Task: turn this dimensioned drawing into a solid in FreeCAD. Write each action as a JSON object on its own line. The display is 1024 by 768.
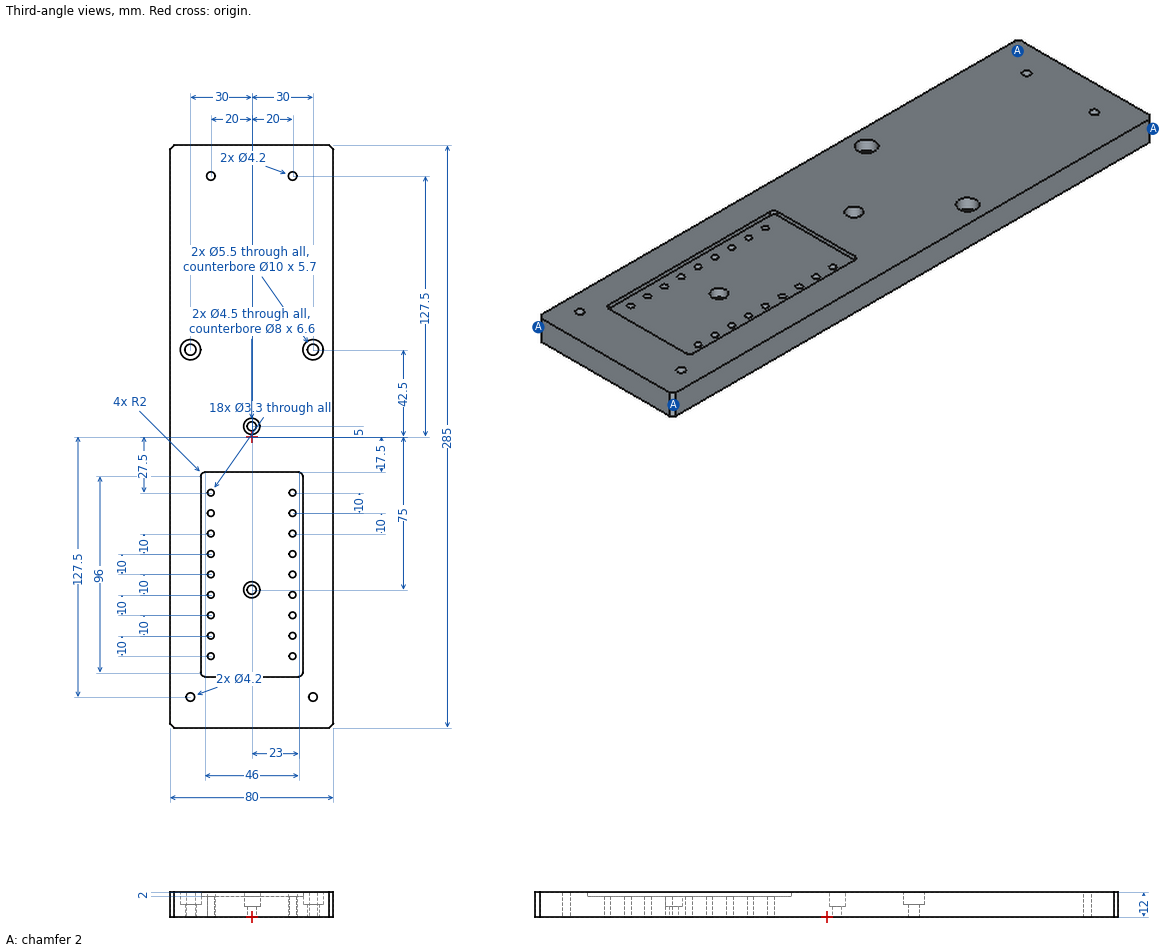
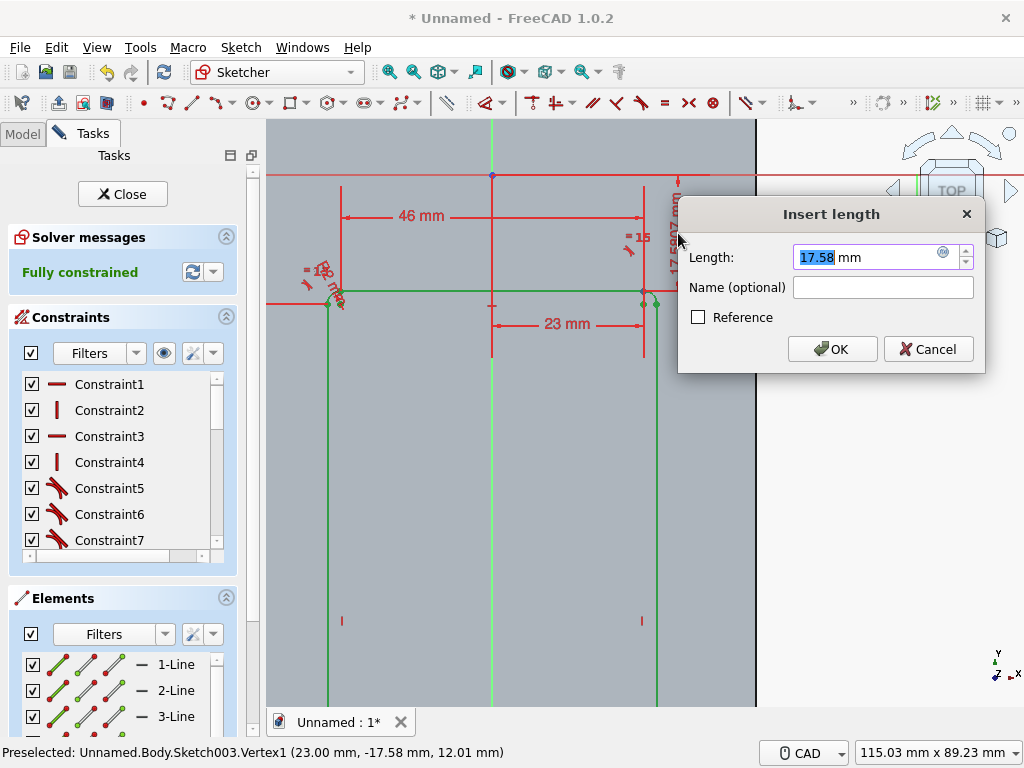
{"action": "type", "text": "17.5"}
{"action": "key", "text": "Return"}
{"action": "key", "text": "Escape"}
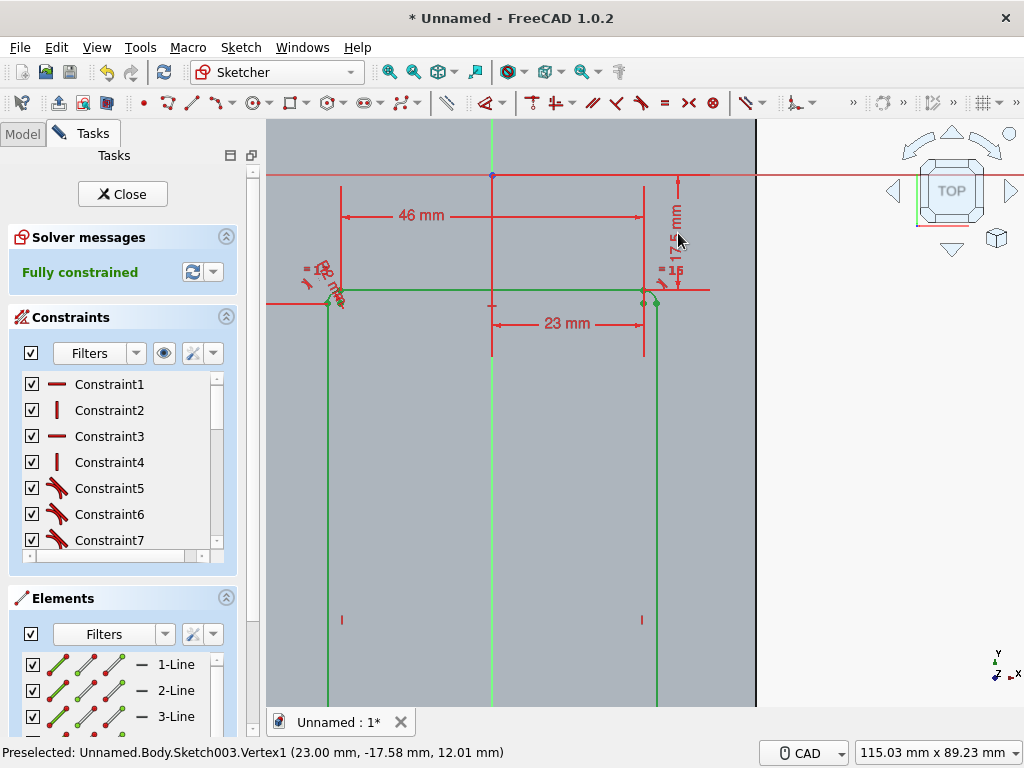
{"action": "left_click", "coordinate": [123, 194]}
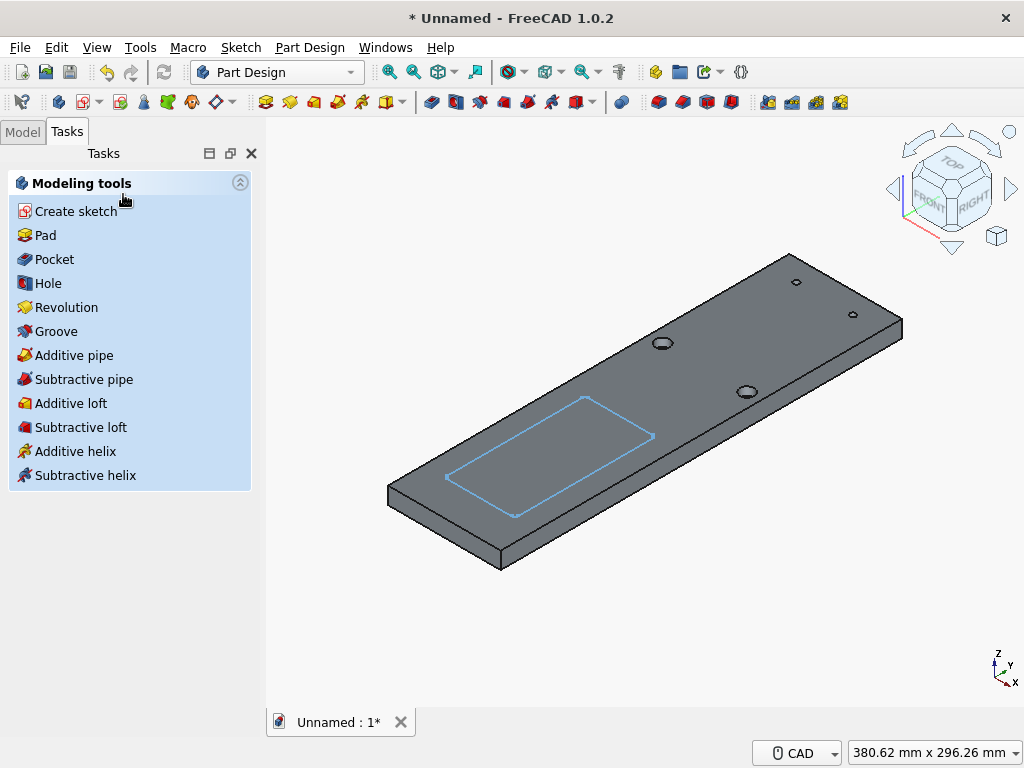
{"action": "left_click", "coordinate": [432, 102]}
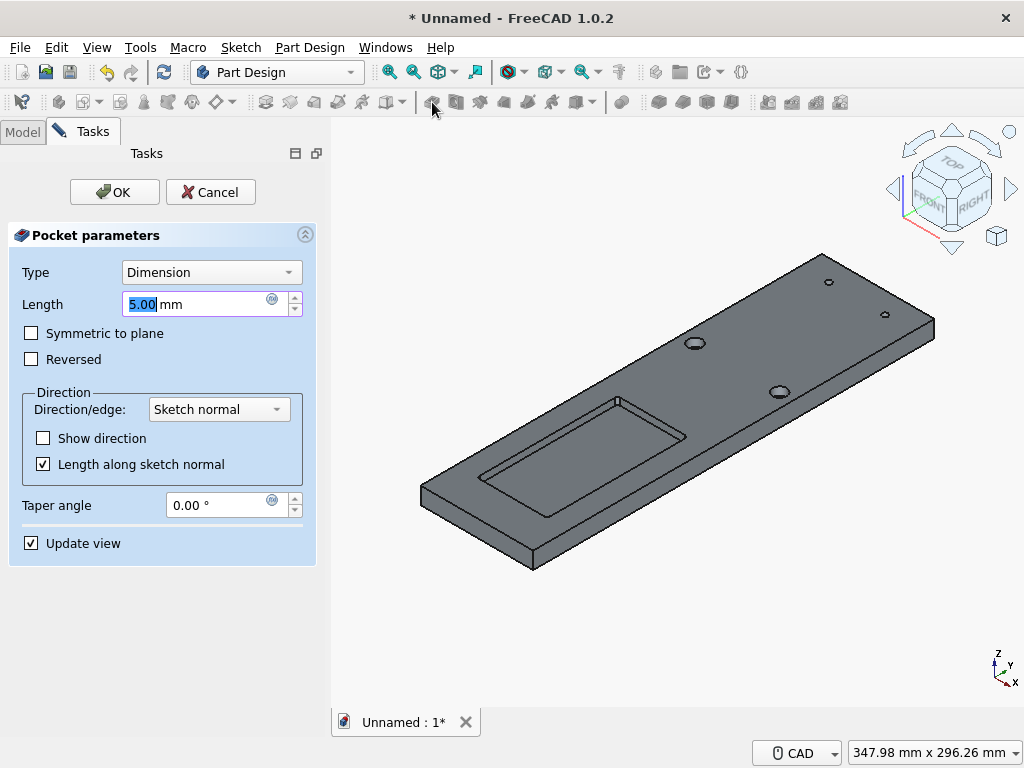
{"action": "type", "text": "2"}
{"action": "key", "text": "Tab"}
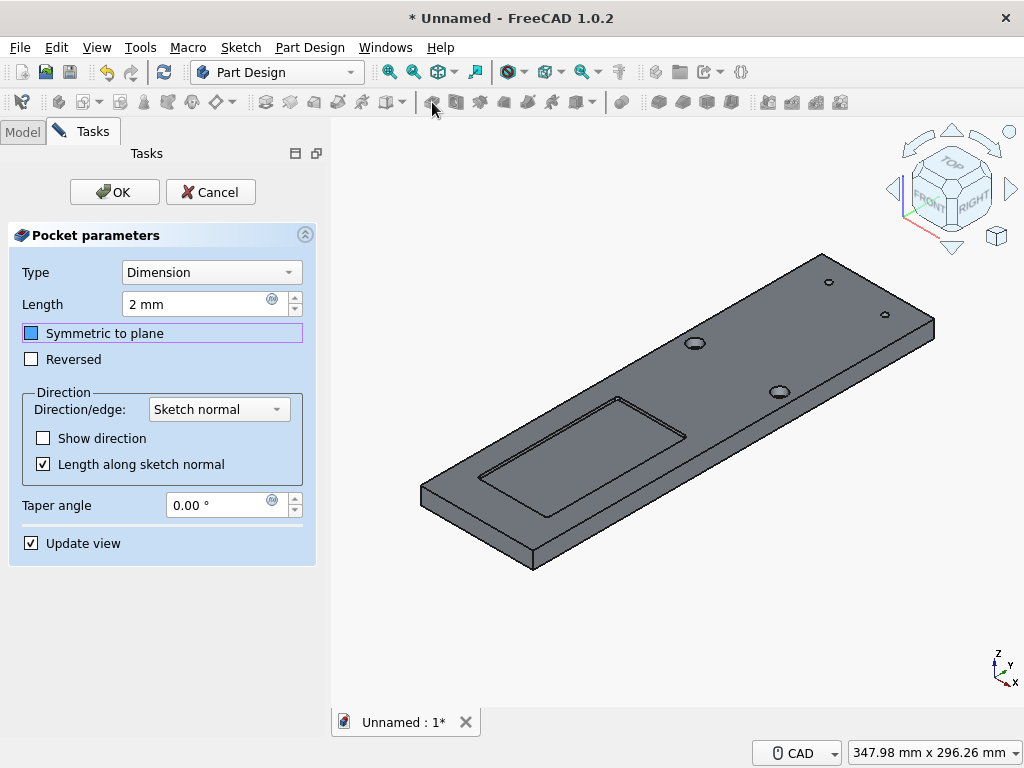
{"action": "left_click", "coordinate": [115, 192]}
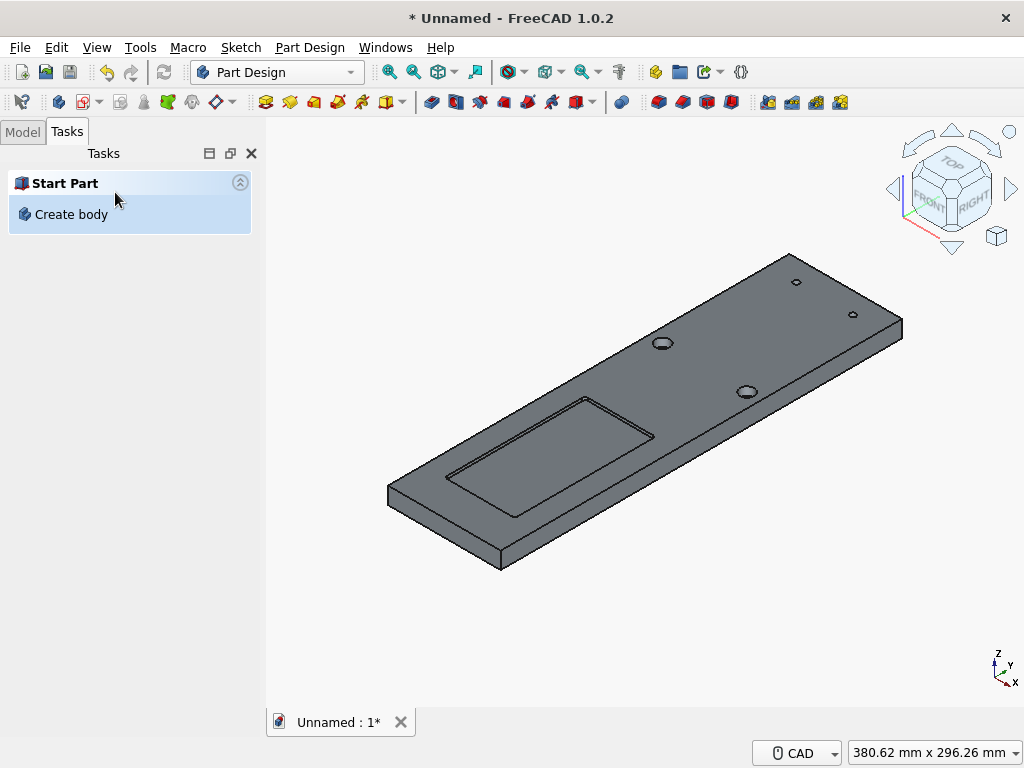
{"action": "left_click", "coordinate": [570, 448]}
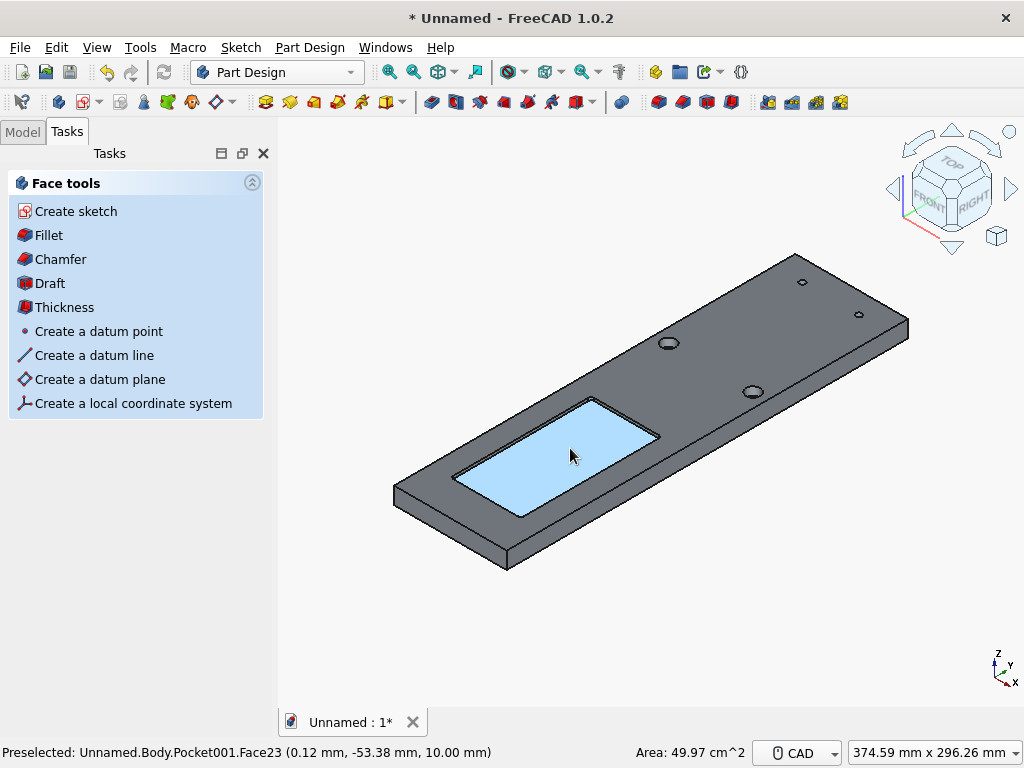
{"action": "left_click", "coordinate": [84, 102]}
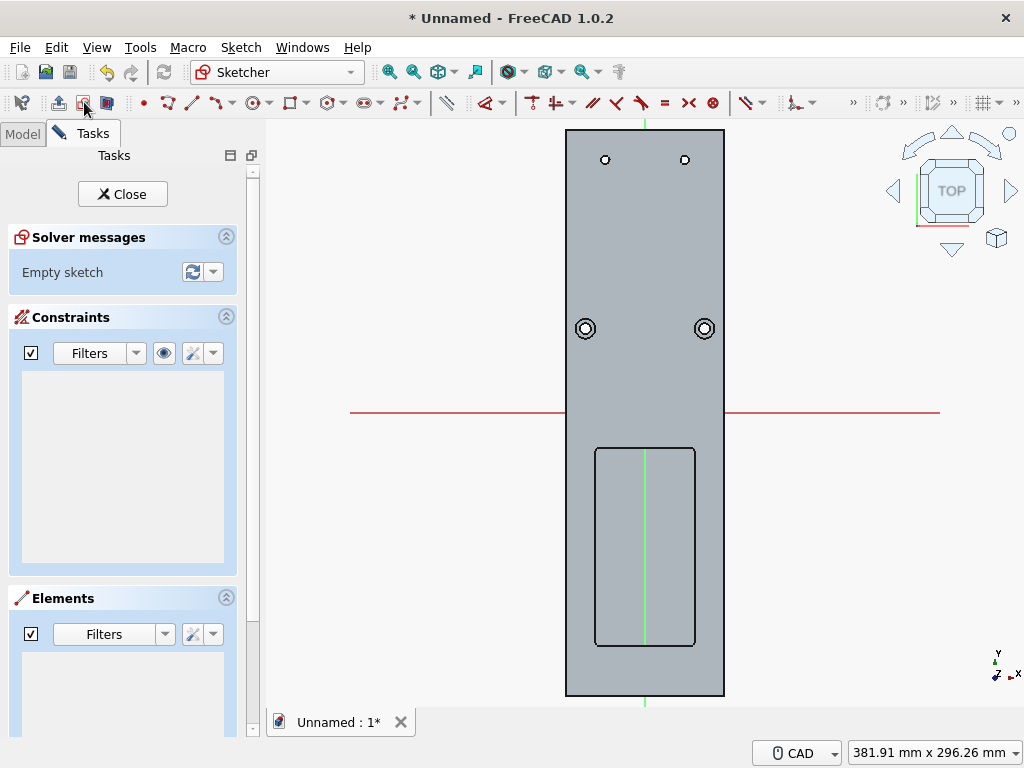
{"action": "key", "text": "q s"}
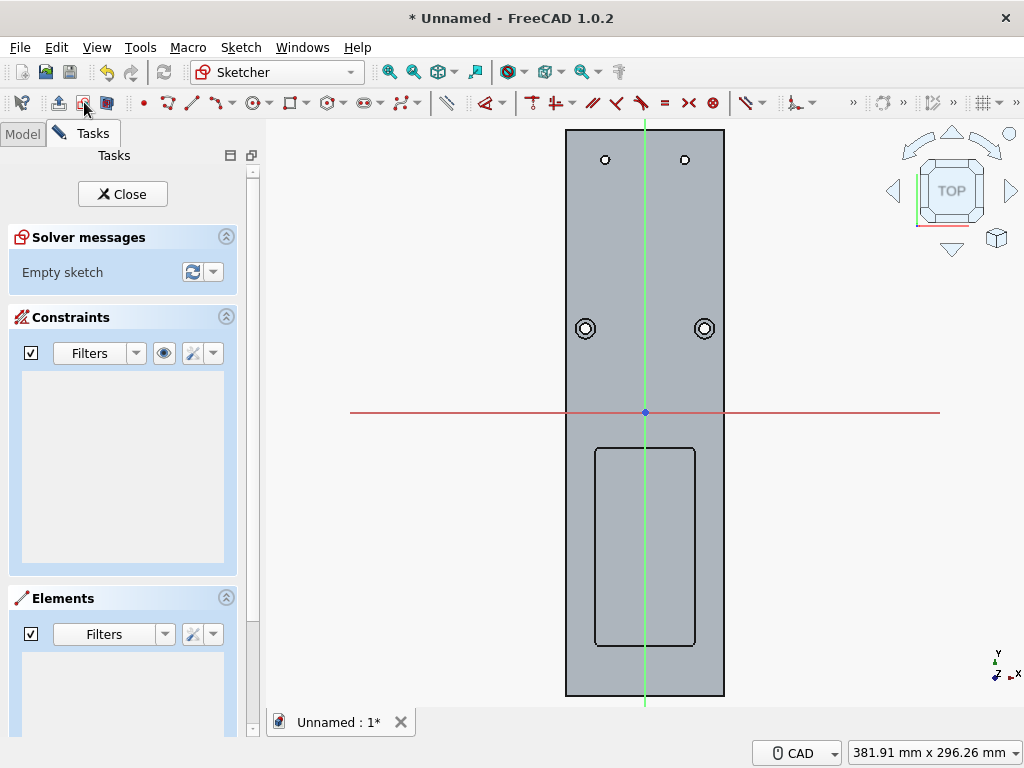
{"action": "scroll", "coordinate": [728, 653], "scroll_direction": "up", "scroll_amount": 3}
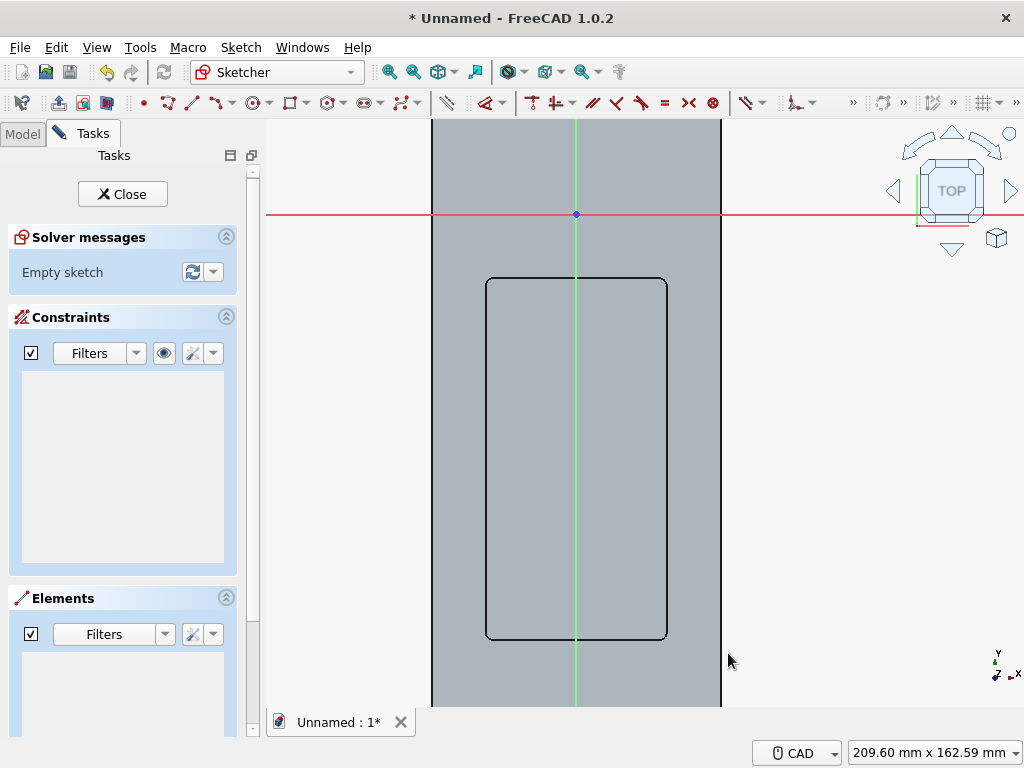
{"action": "key", "text": "g c"}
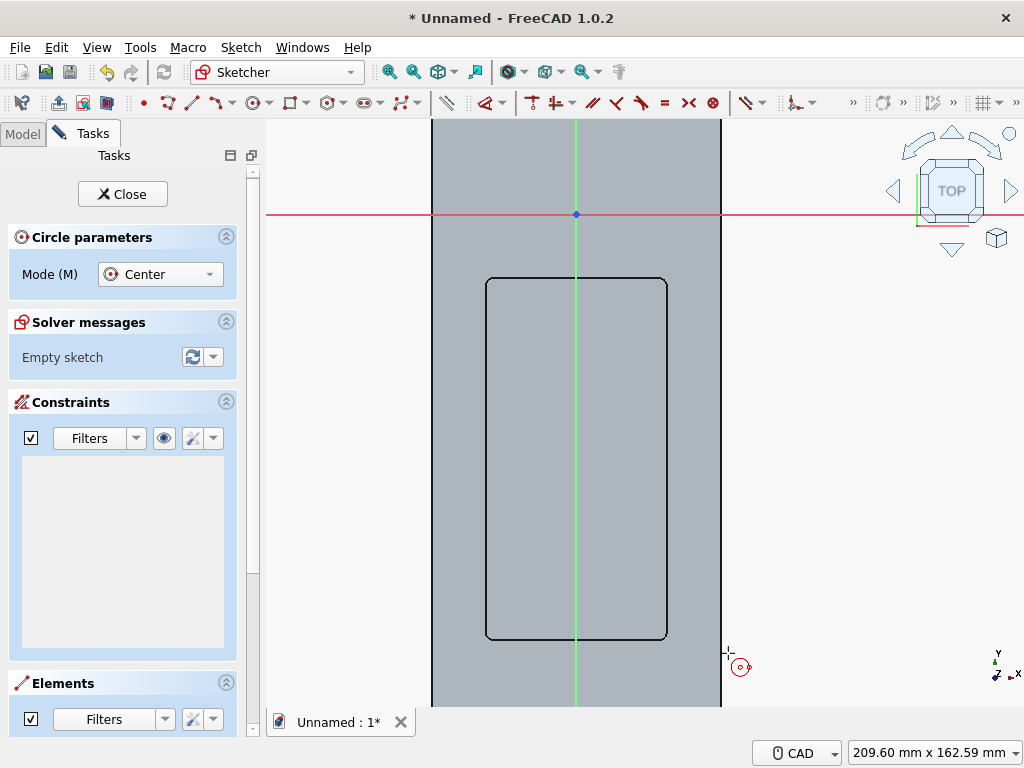
{"action": "scroll", "coordinate": [504, 314], "scroll_direction": "up", "scroll_amount": 7}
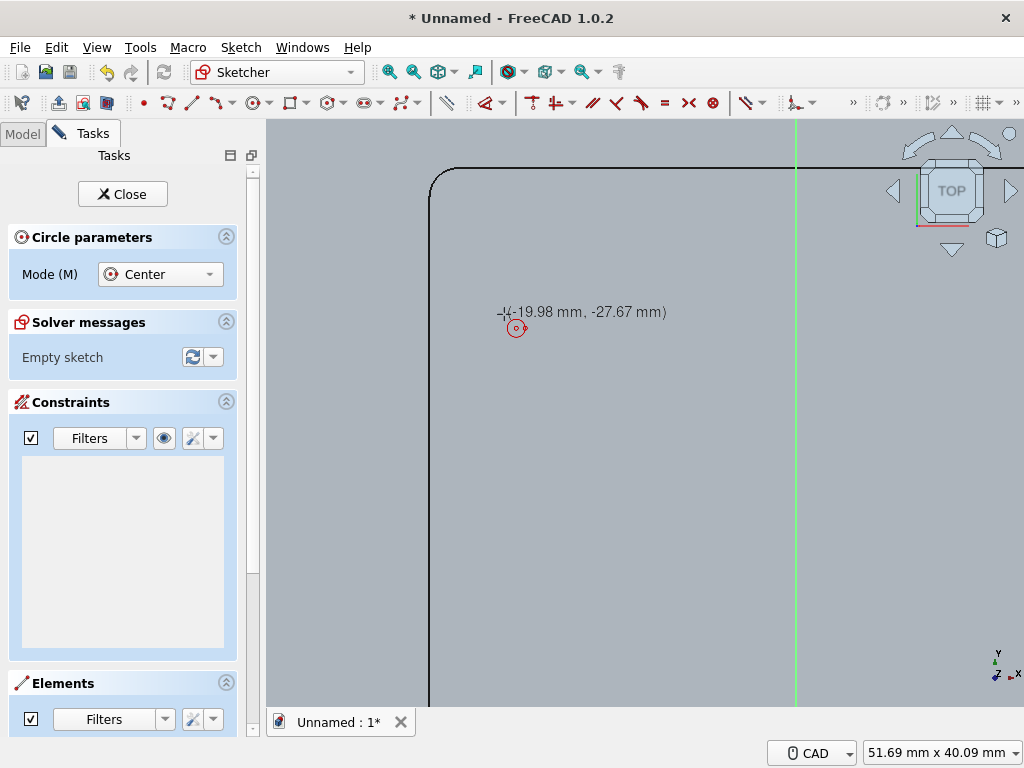
{"action": "scroll", "coordinate": [505, 315], "scroll_direction": "down", "scroll_amount": 7}